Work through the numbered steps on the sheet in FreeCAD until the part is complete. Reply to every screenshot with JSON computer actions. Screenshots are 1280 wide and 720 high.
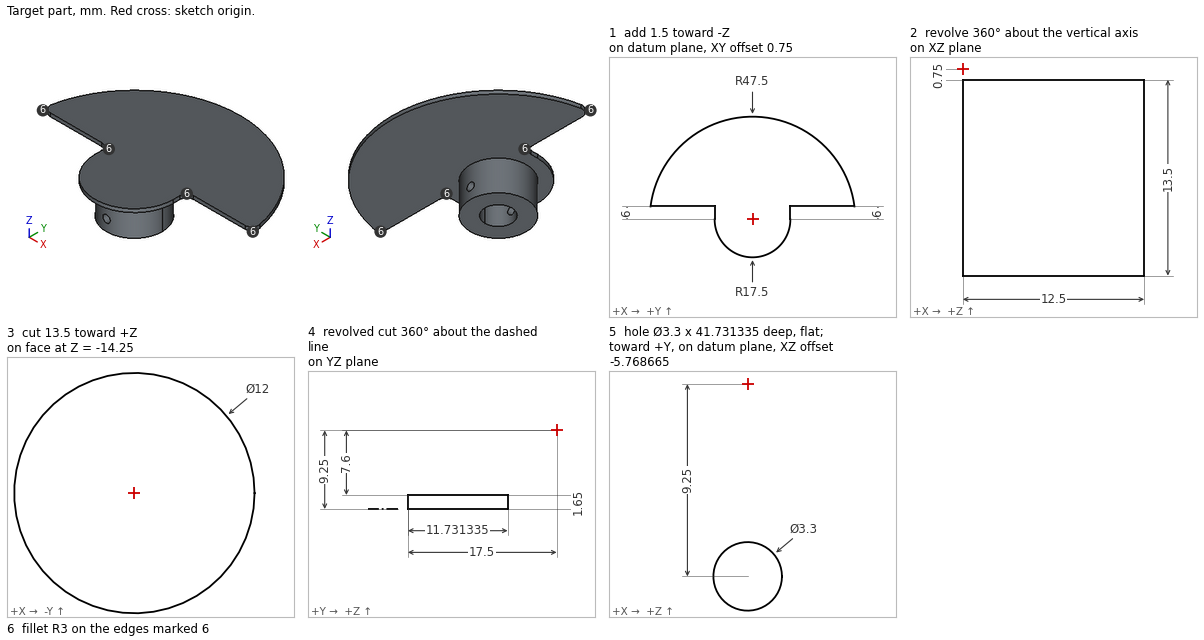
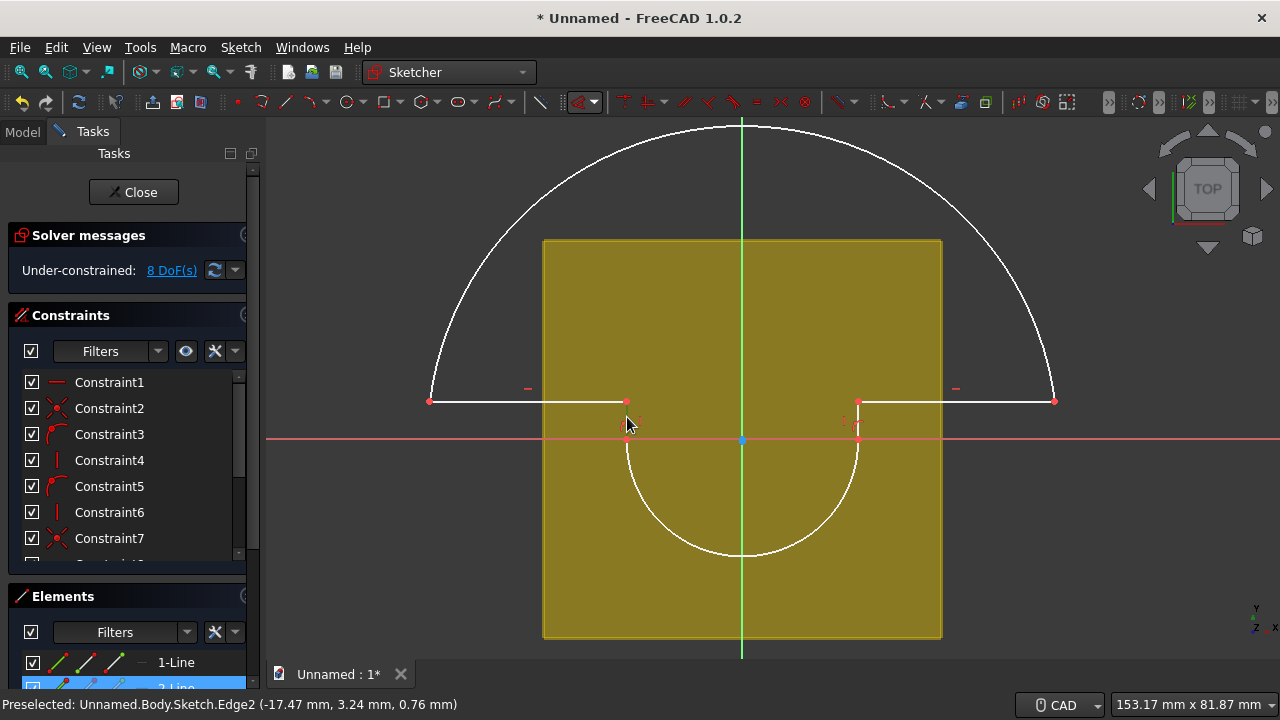
{"action": "left_click", "coordinate": [674, 534]}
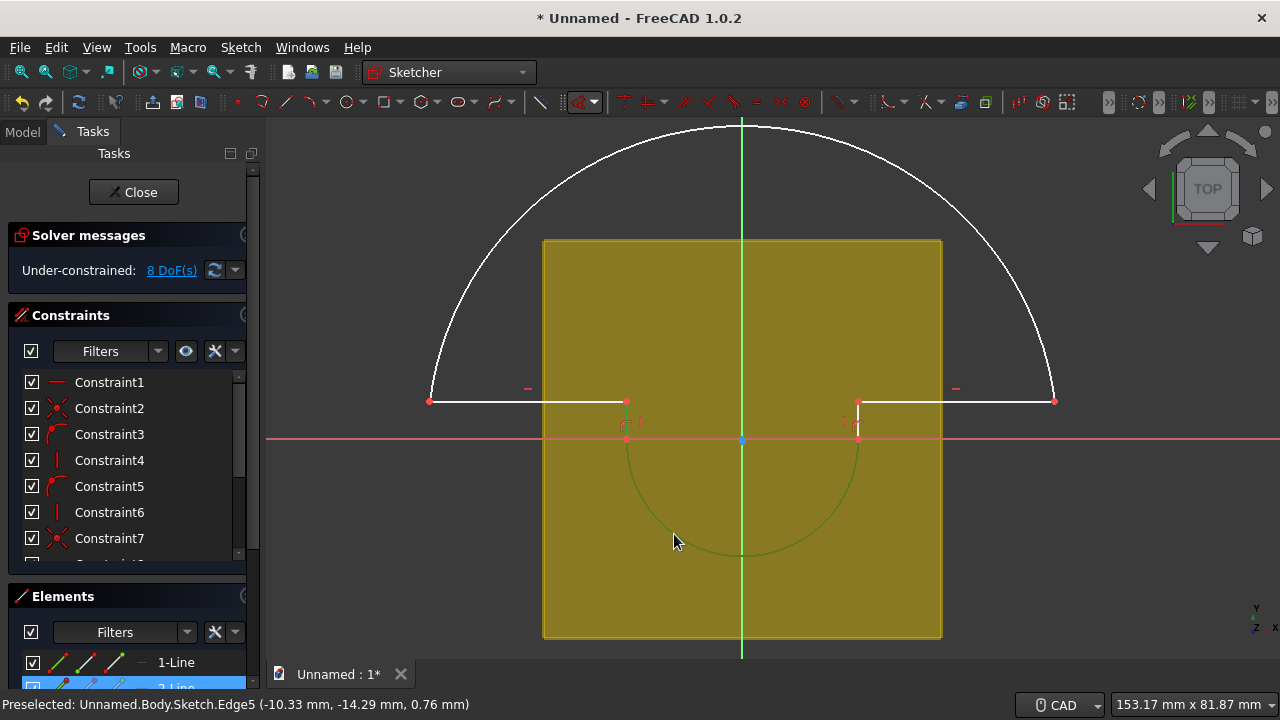
{"action": "key", "text": "t"}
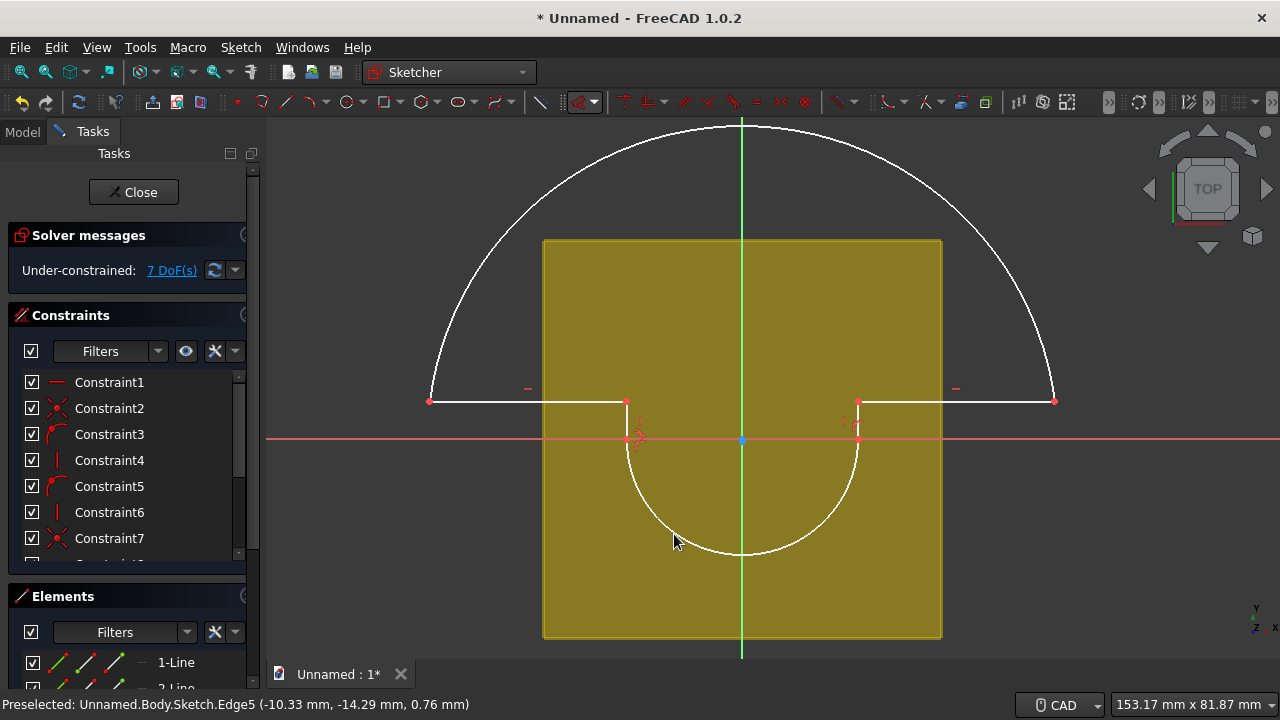
{"action": "left_click", "coordinate": [674, 533]}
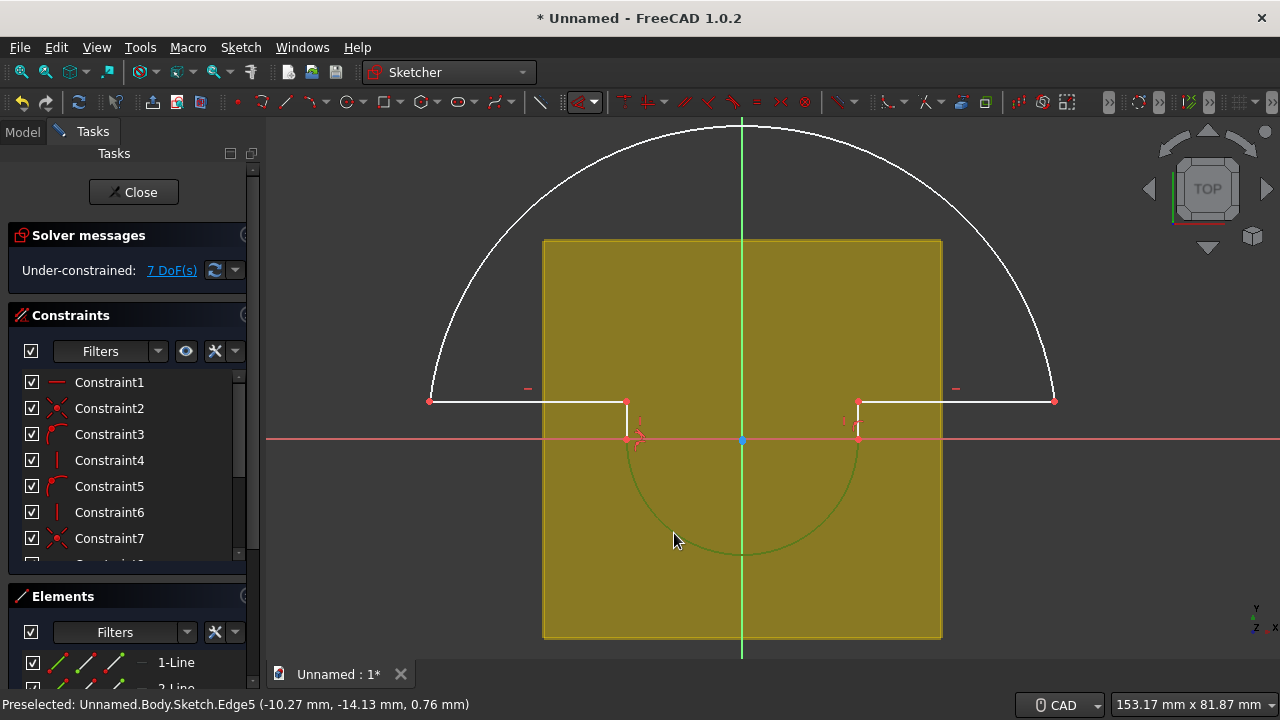
{"action": "left_click", "coordinate": [915, 177]}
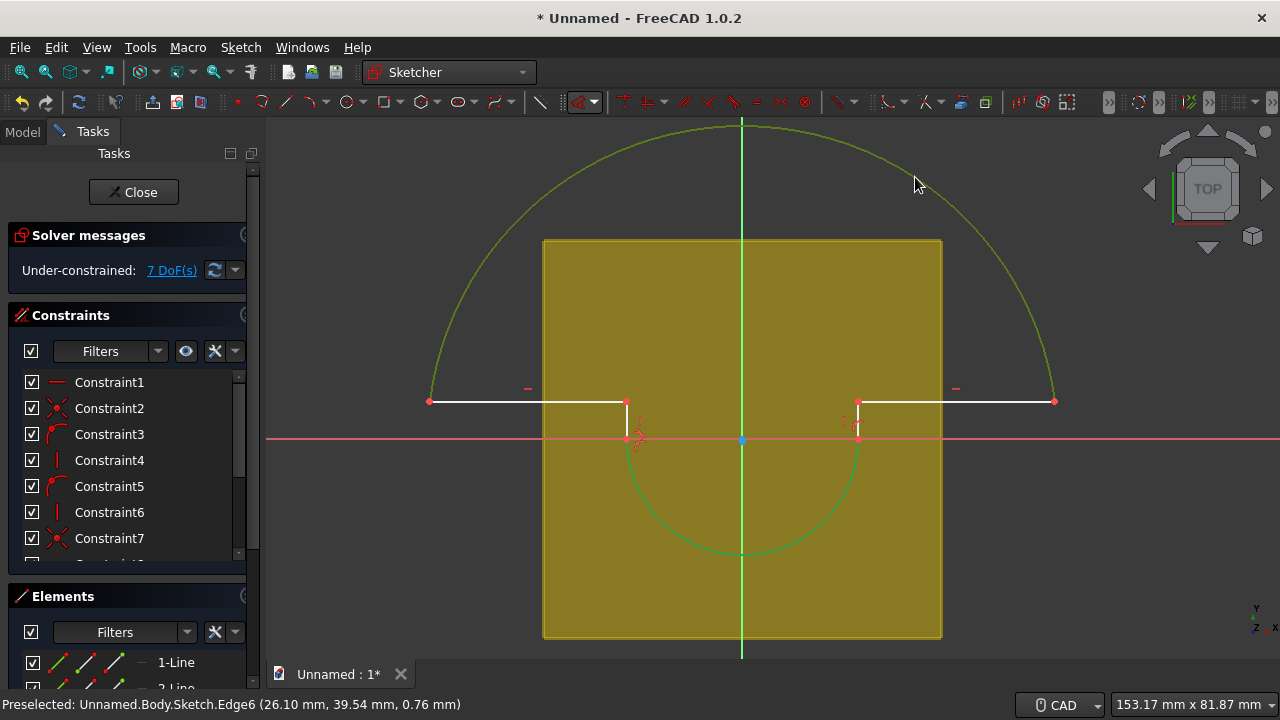
{"action": "key", "text": "c"}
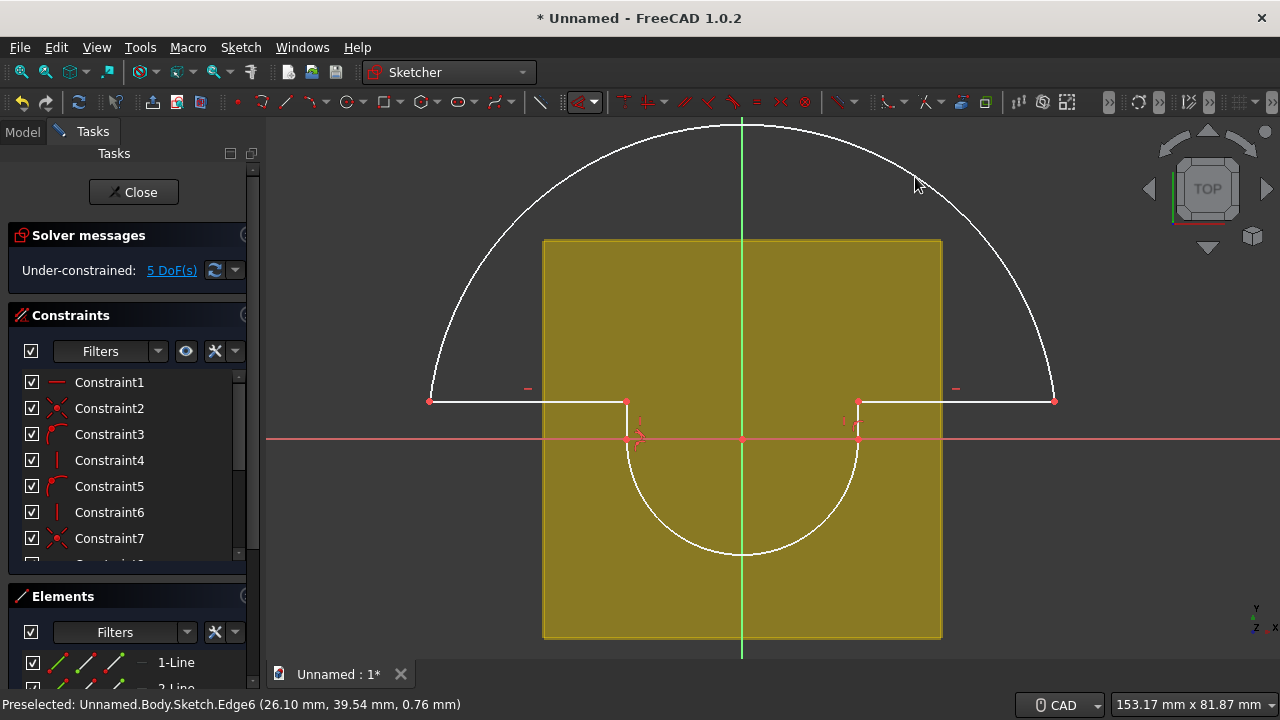
{"action": "left_click", "coordinate": [742, 439]}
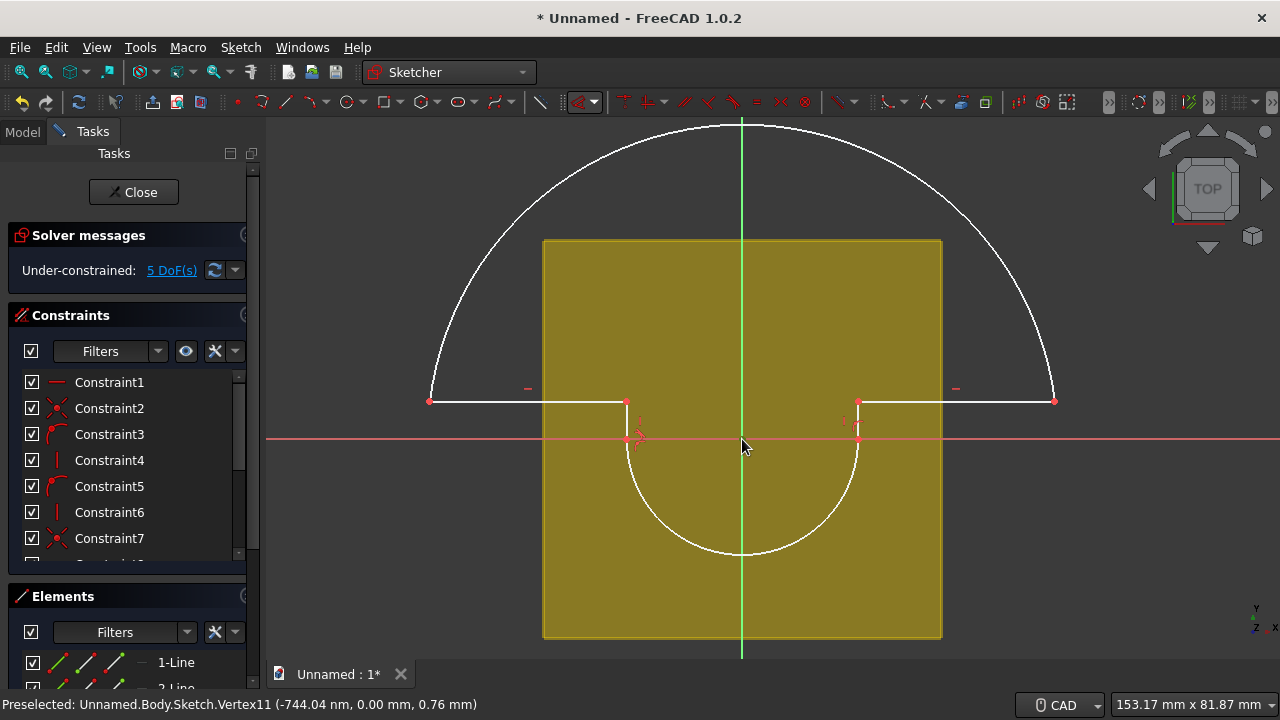
{"action": "left_click", "coordinate": [742, 596]}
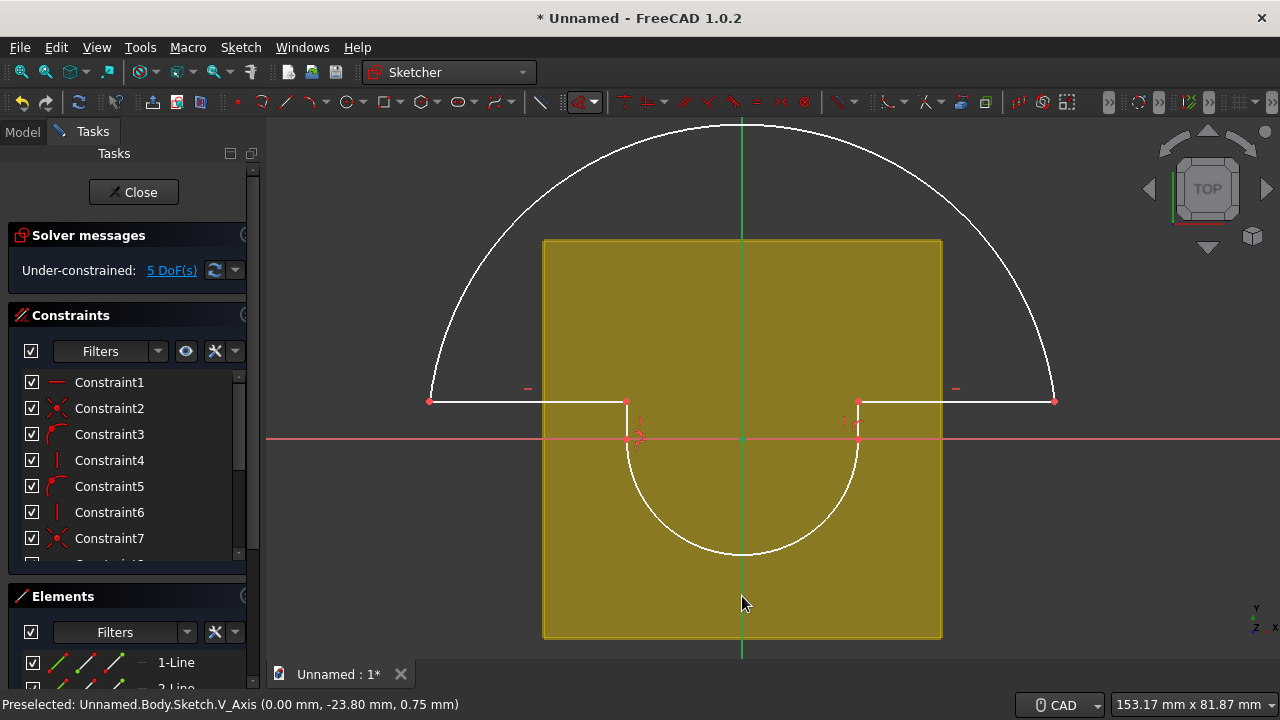
{"action": "key", "text": "c"}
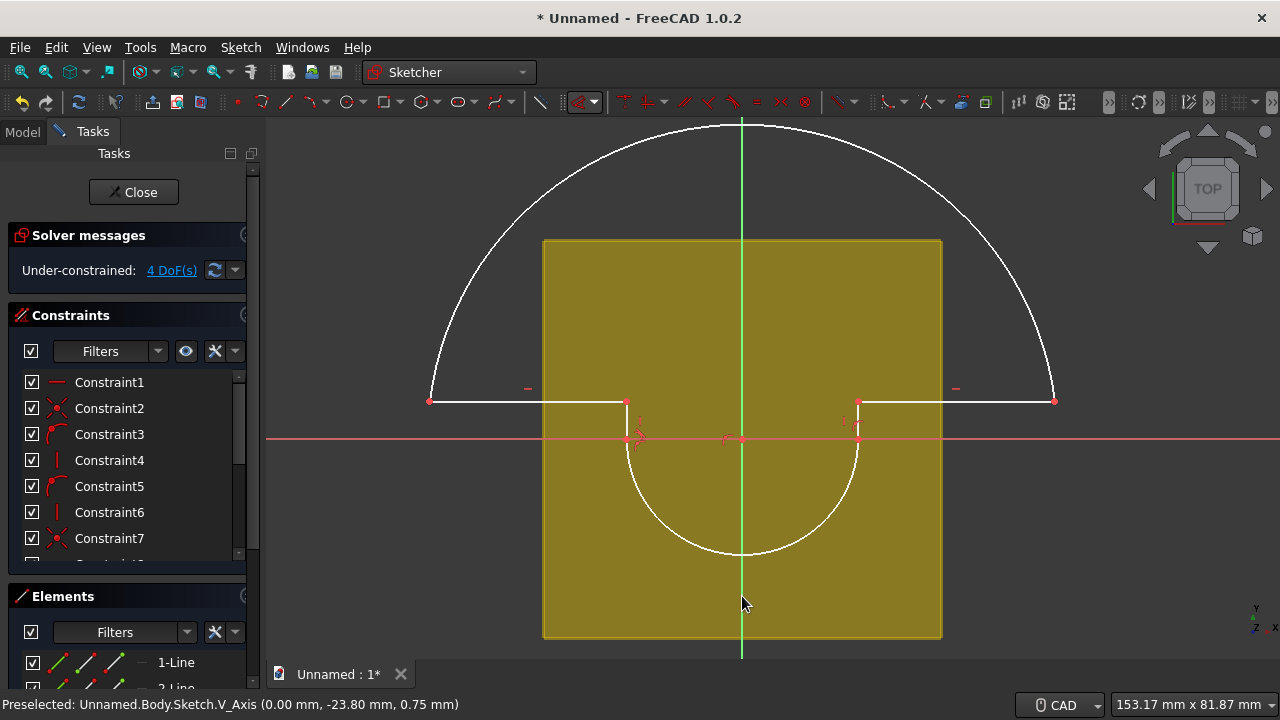
{"action": "key", "text": "d"}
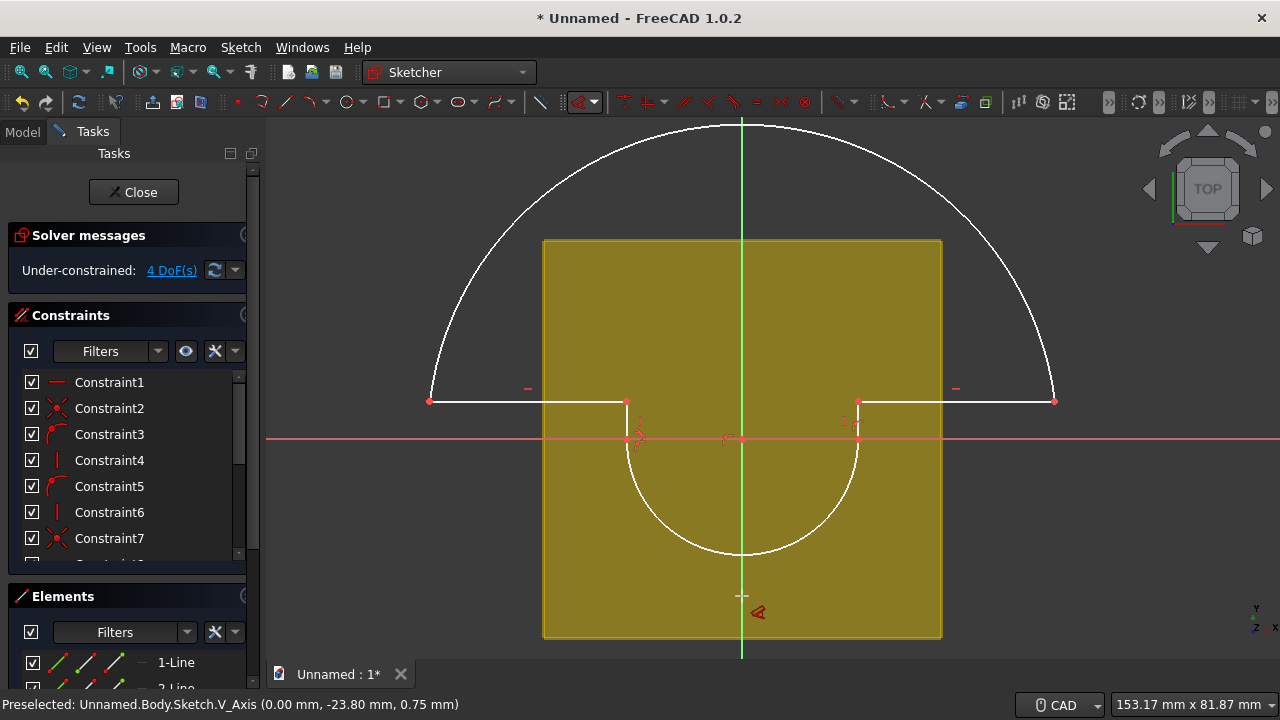
{"action": "left_click", "coordinate": [674, 533]}
{"action": "left_click", "coordinate": [655, 559]}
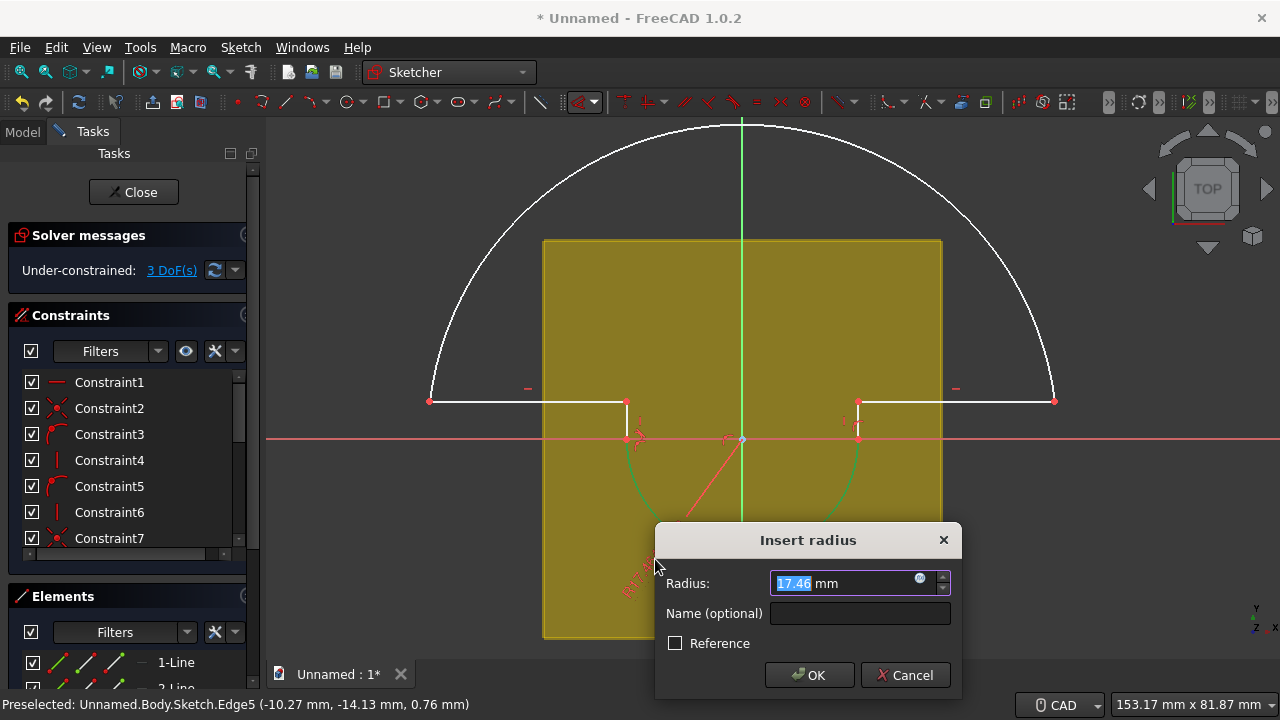
{"action": "type", "text": "17.5"}
{"action": "key", "text": "Return"}